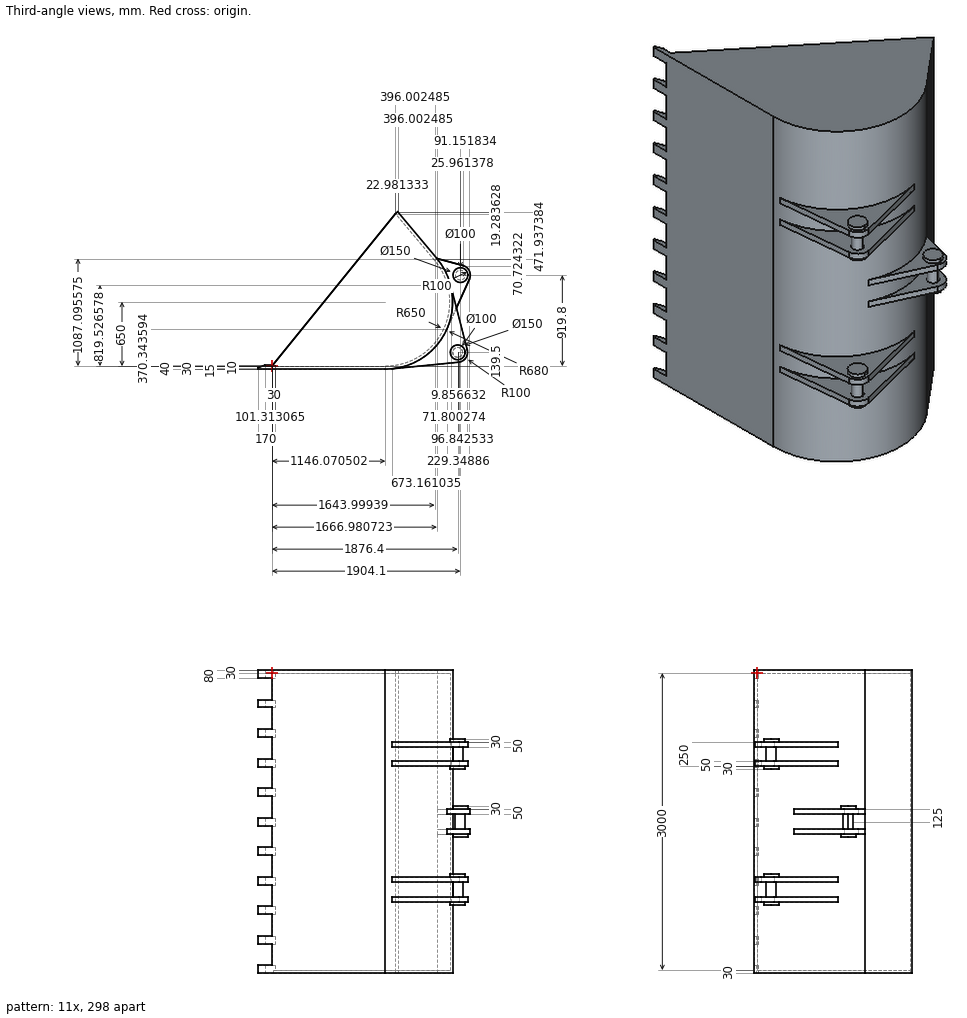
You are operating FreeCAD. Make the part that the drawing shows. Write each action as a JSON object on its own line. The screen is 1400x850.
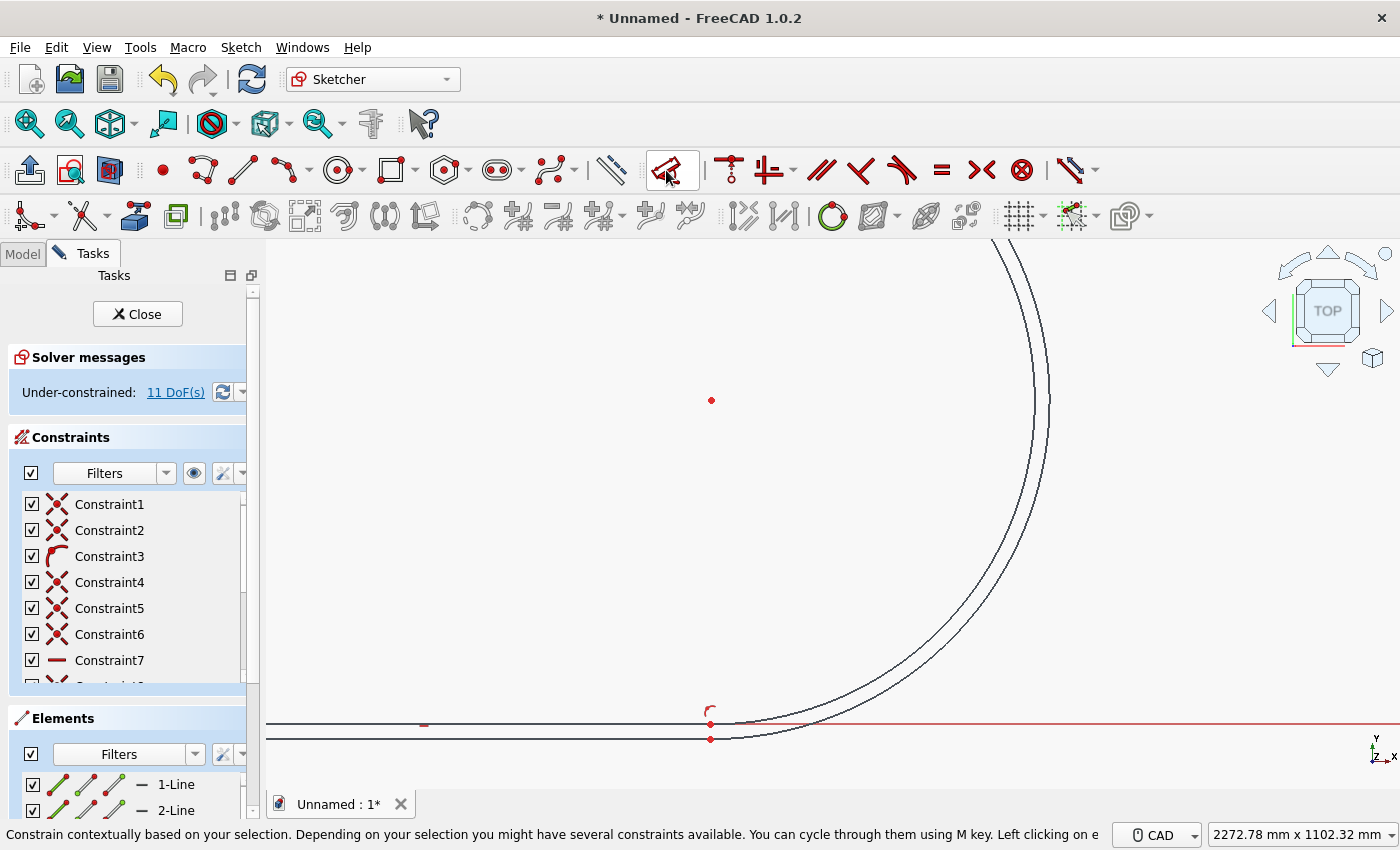
{"action": "left_click", "coordinate": [915, 653]}
{"action": "left_click", "coordinate": [935, 678]}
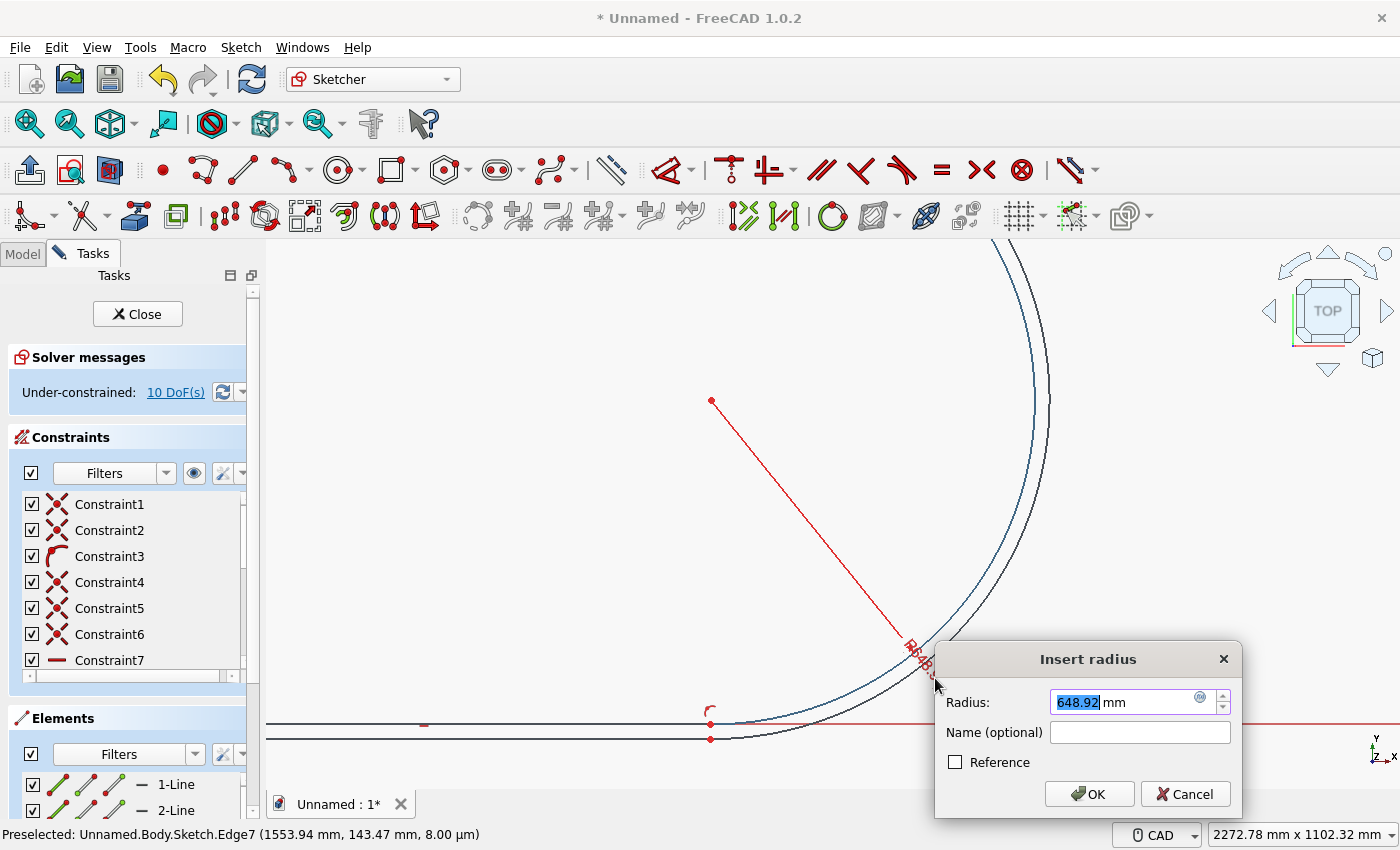
{"action": "type", "text": "650"}
{"action": "key", "text": "Return"}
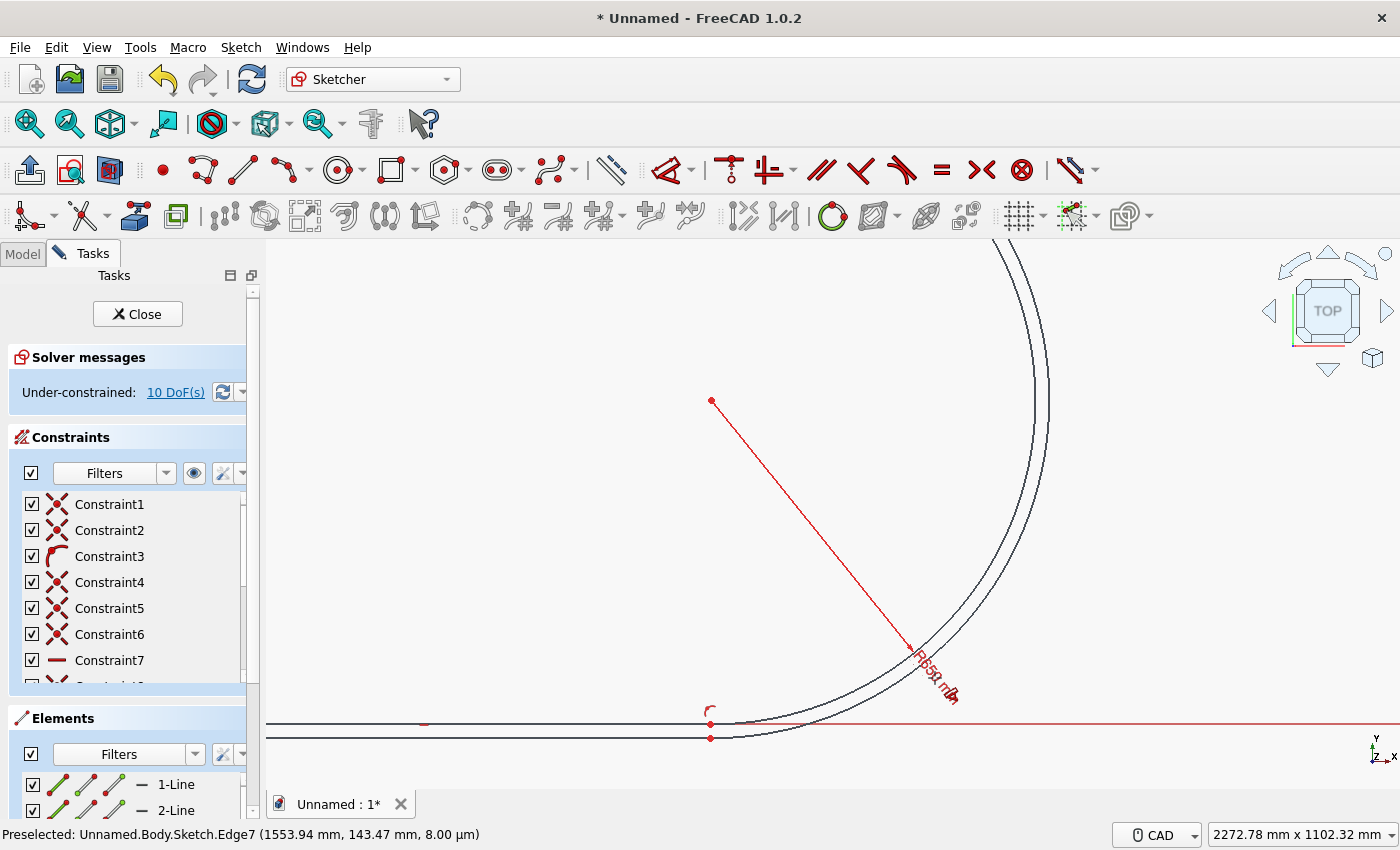
{"action": "left_click", "coordinate": [923, 663]}
{"action": "left_click", "coordinate": [1053, 541]}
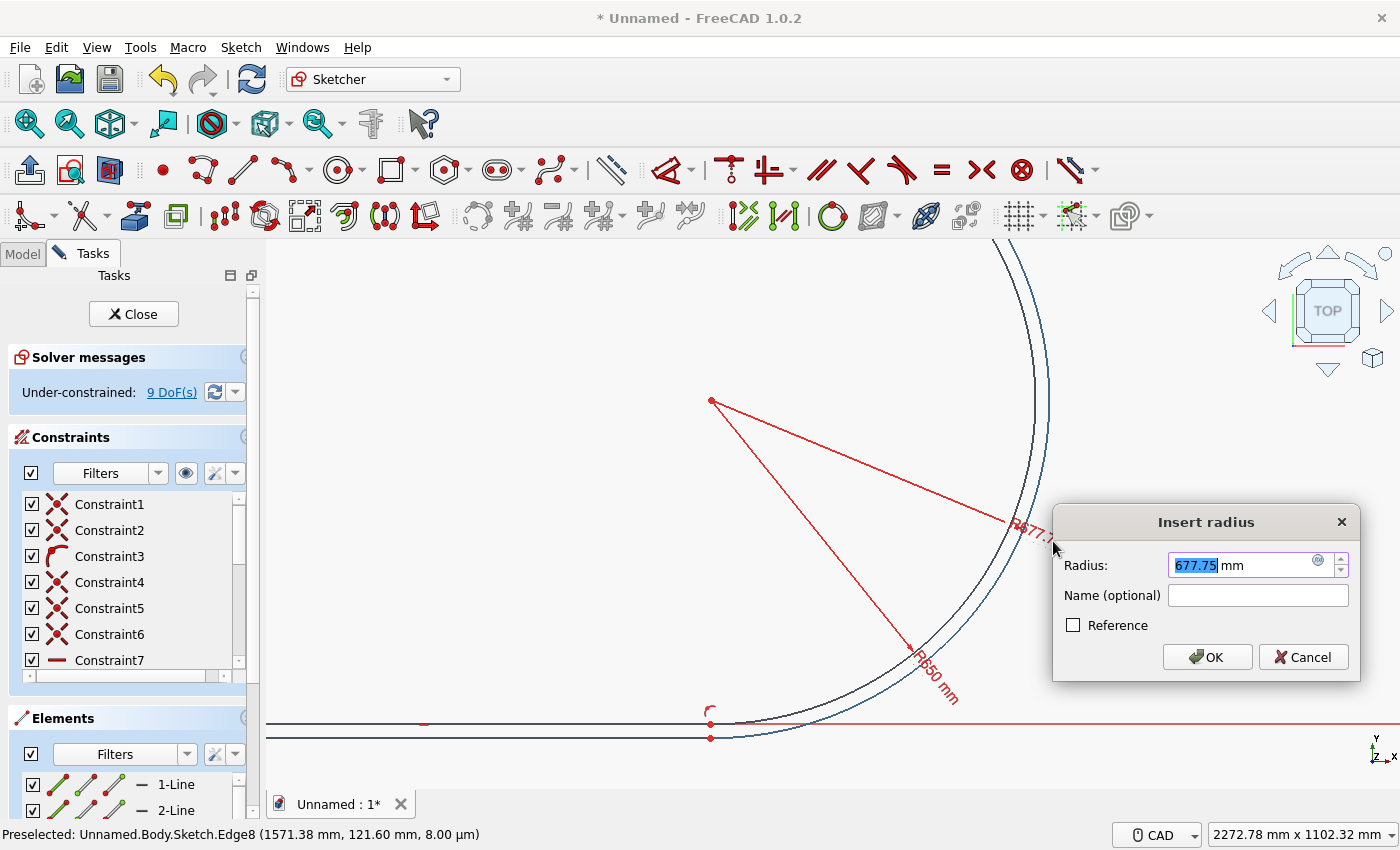
{"action": "type", "text": "680"}
{"action": "key", "text": "Return"}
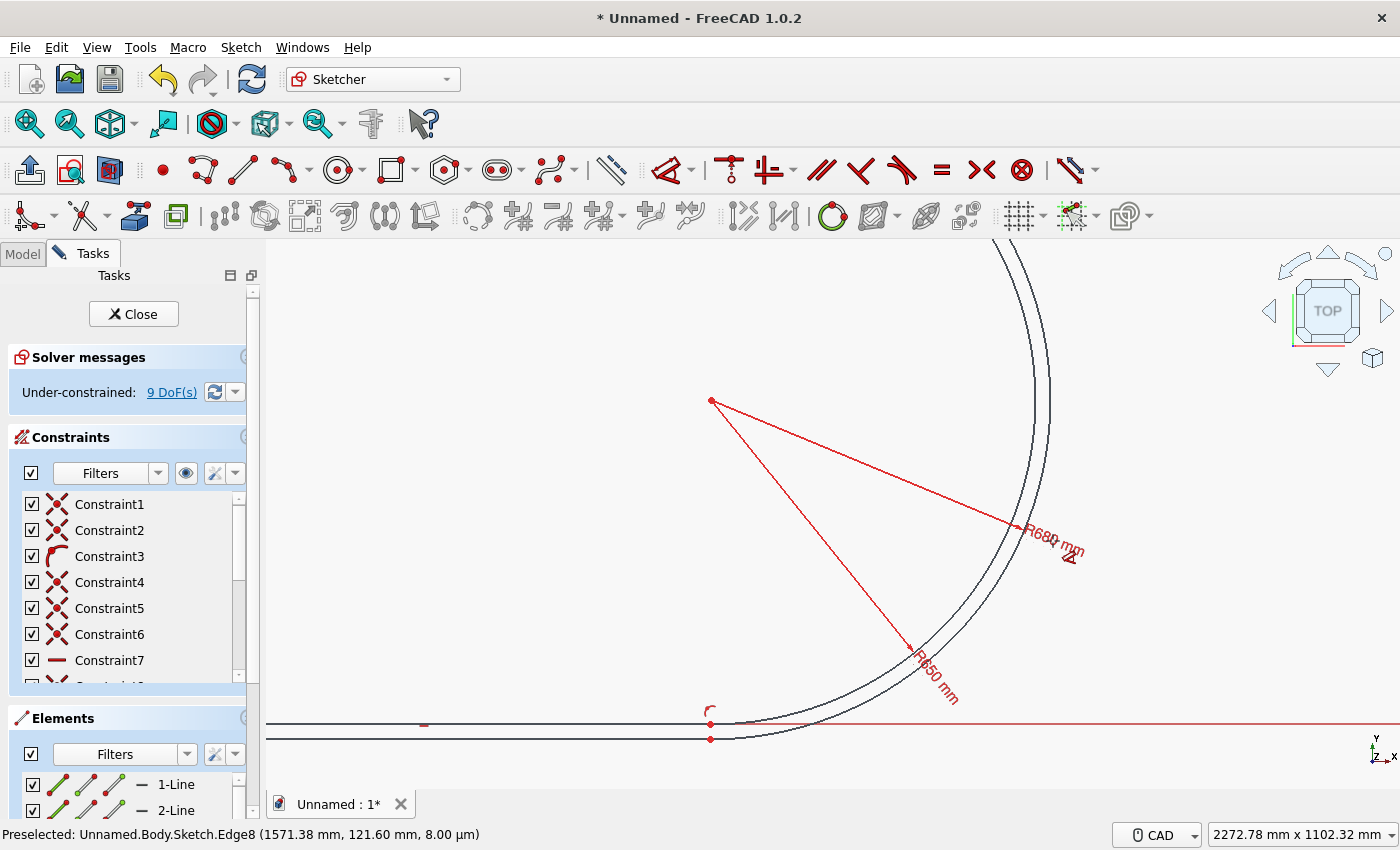
{"action": "scroll", "coordinate": [916, 654], "scroll_direction": "down", "scroll_amount": 4}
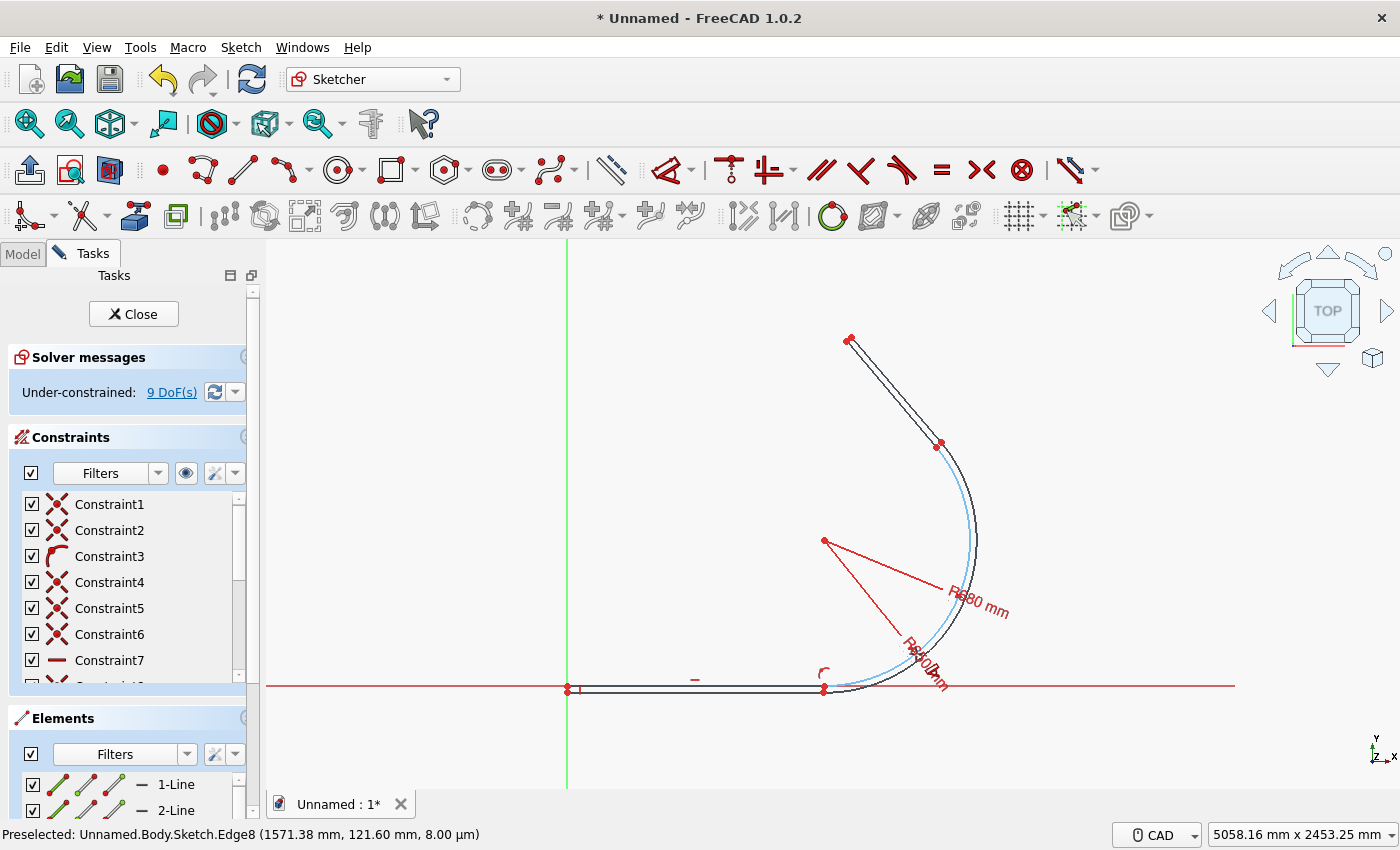
{"action": "scroll", "coordinate": [849, 339], "scroll_direction": "up", "scroll_amount": 11}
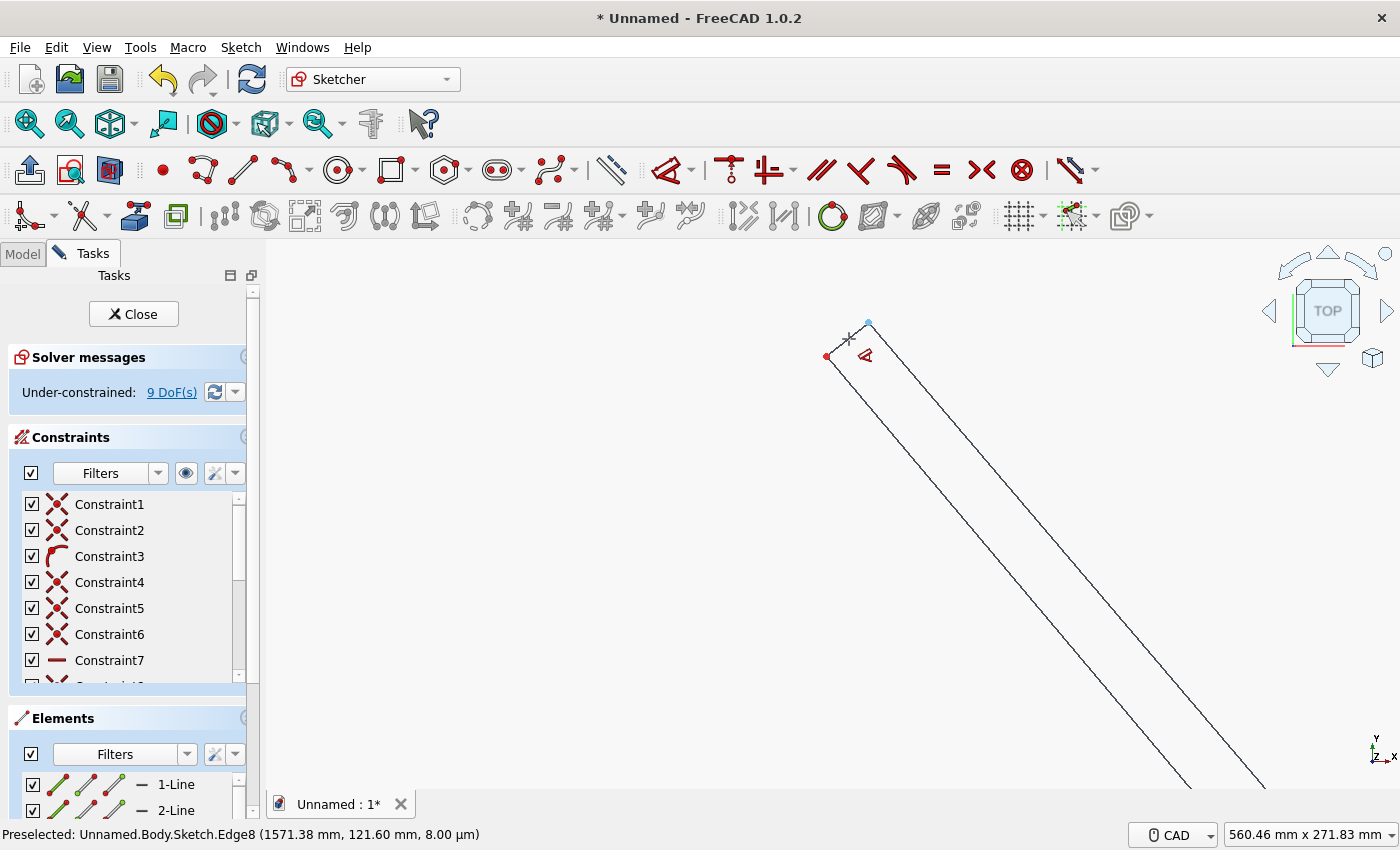
{"action": "left_click", "coordinate": [848, 340]}
{"action": "left_click", "coordinate": [848, 289]}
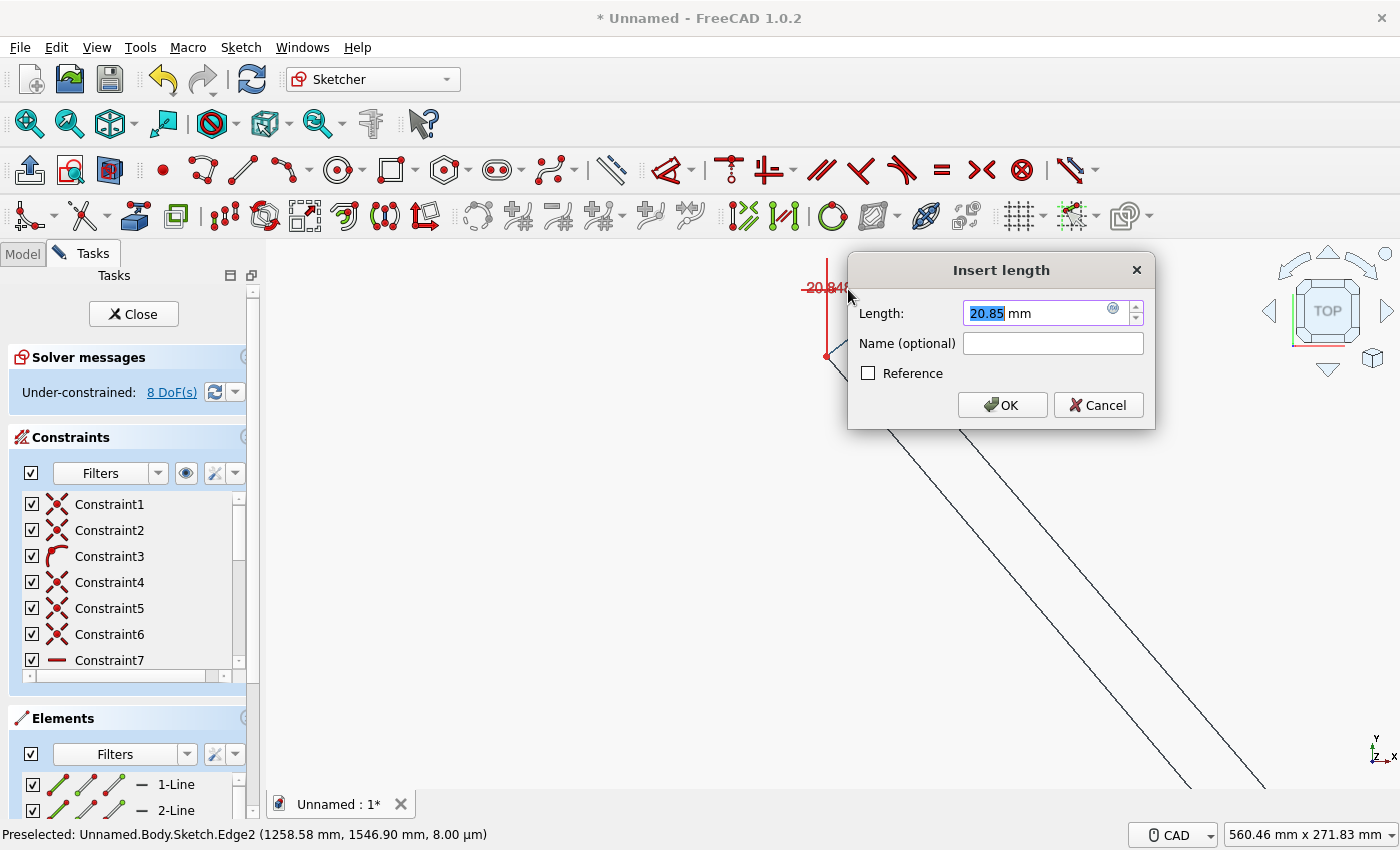
{"action": "type", "text": "22.981333"}
{"action": "key", "text": "Return"}